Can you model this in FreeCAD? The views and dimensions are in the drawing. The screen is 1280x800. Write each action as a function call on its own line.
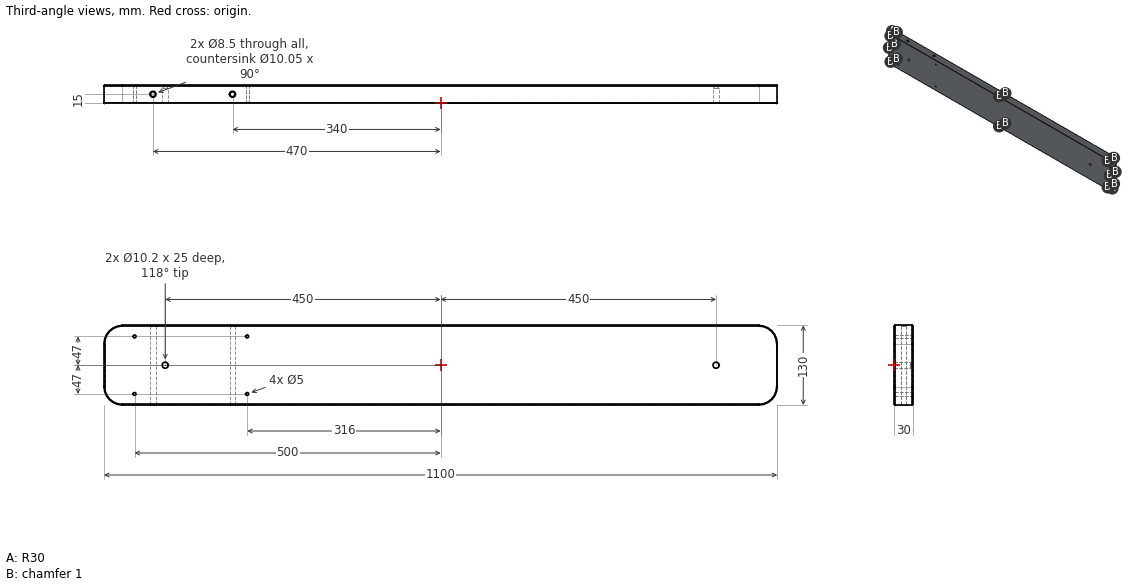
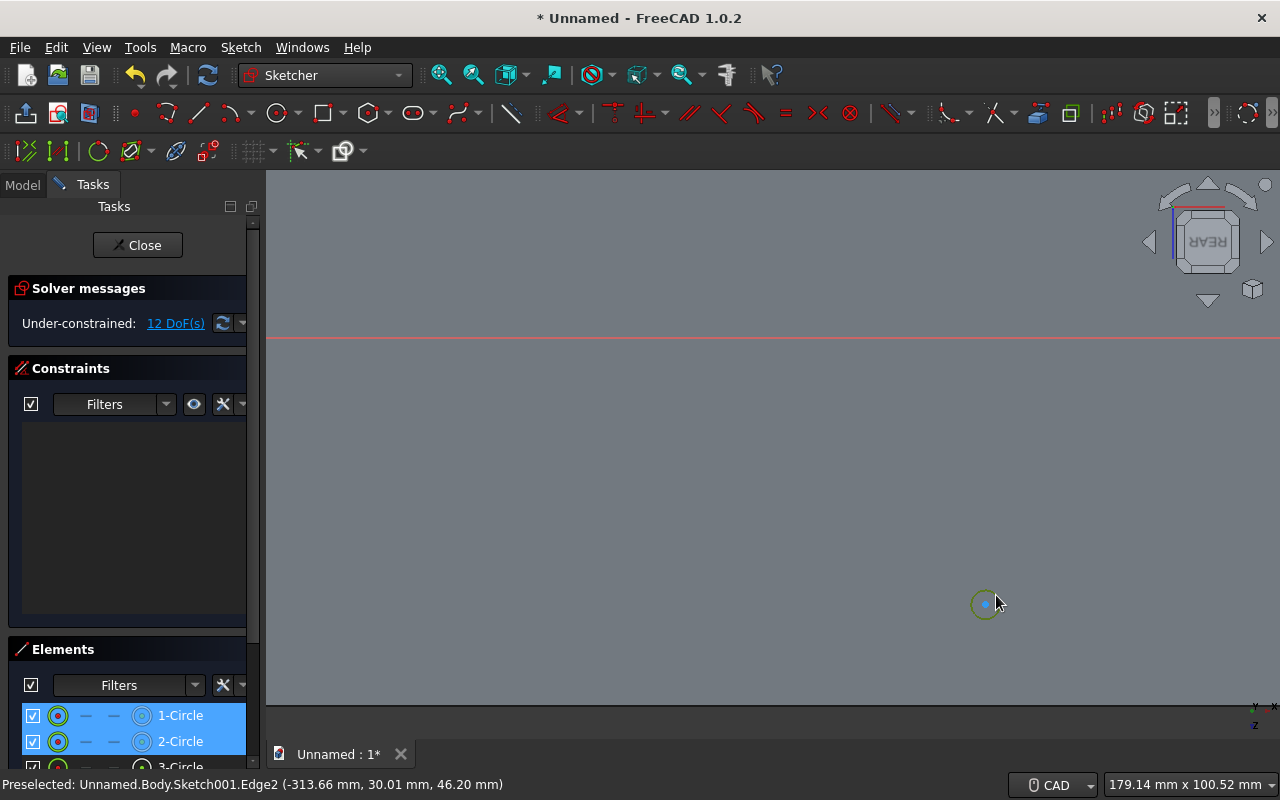
scroll(996, 596, down, 3)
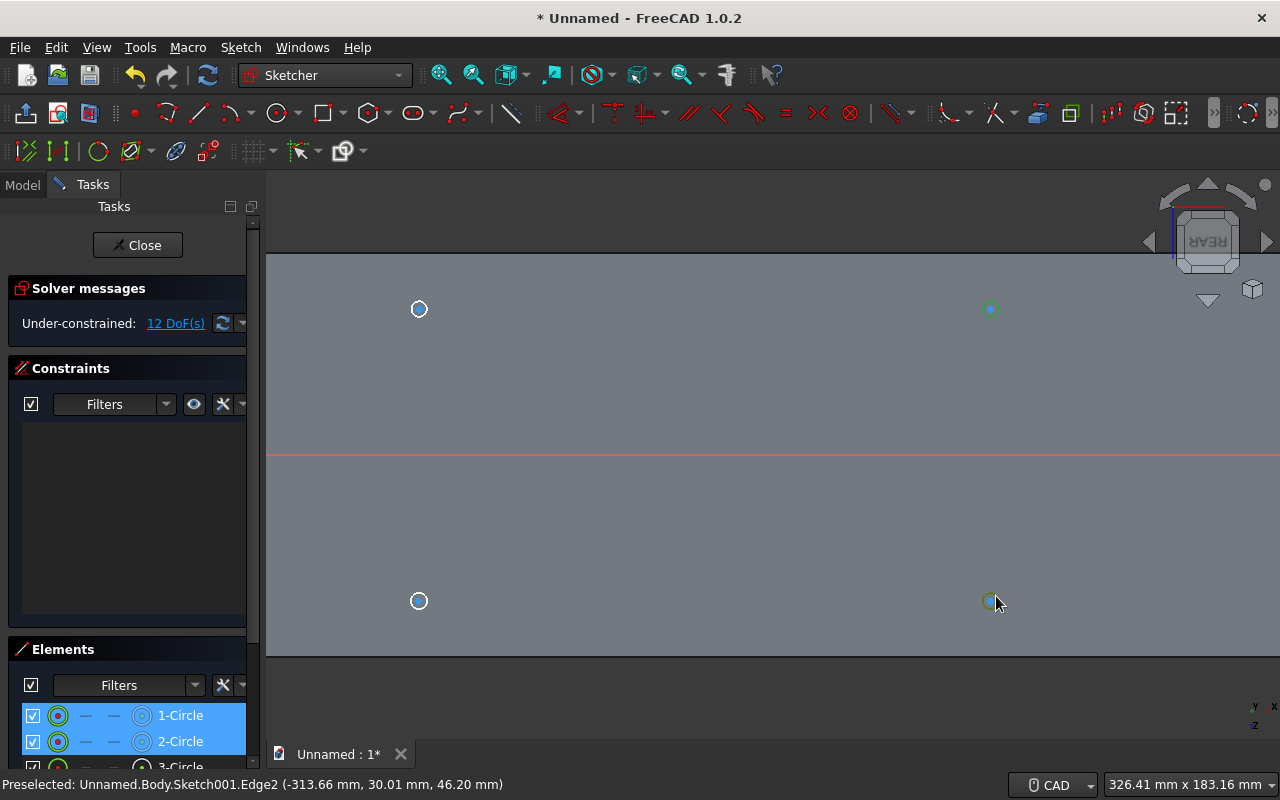
scroll(425, 304, up, 3)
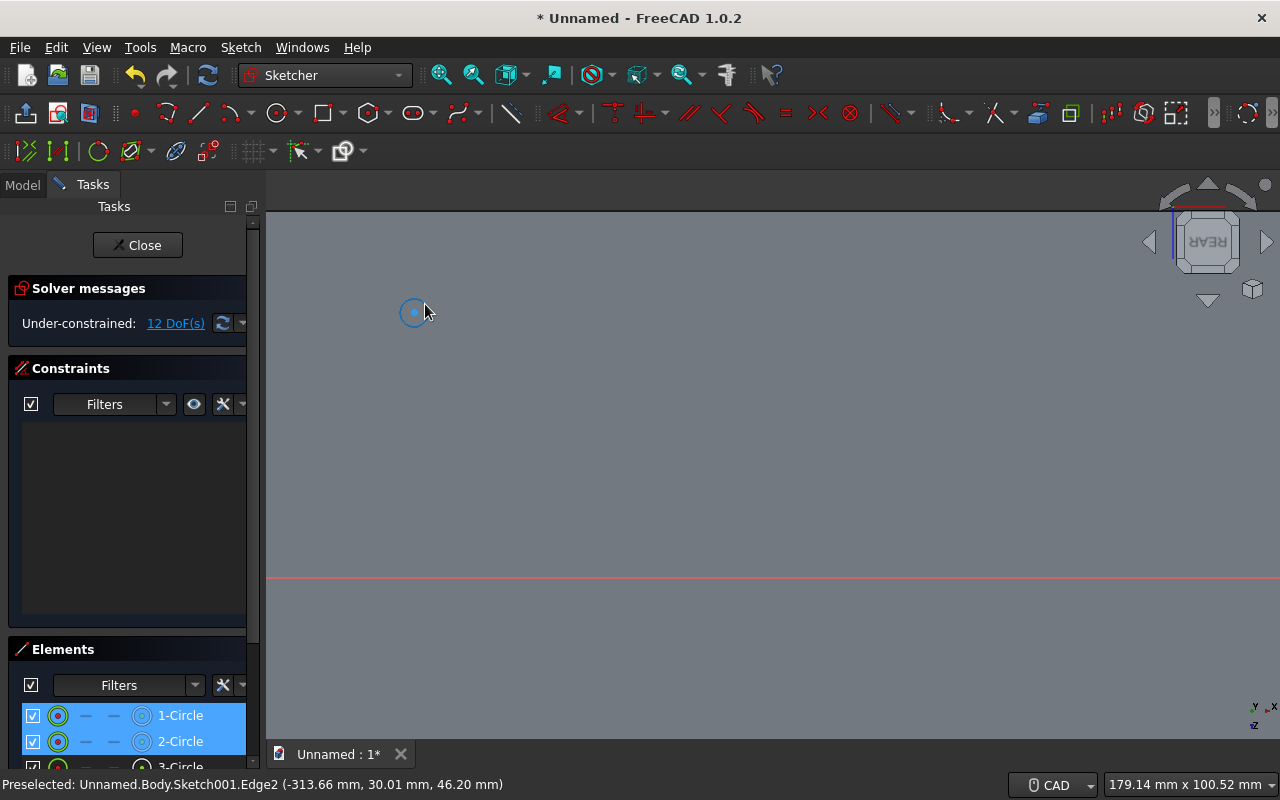
click(424, 303)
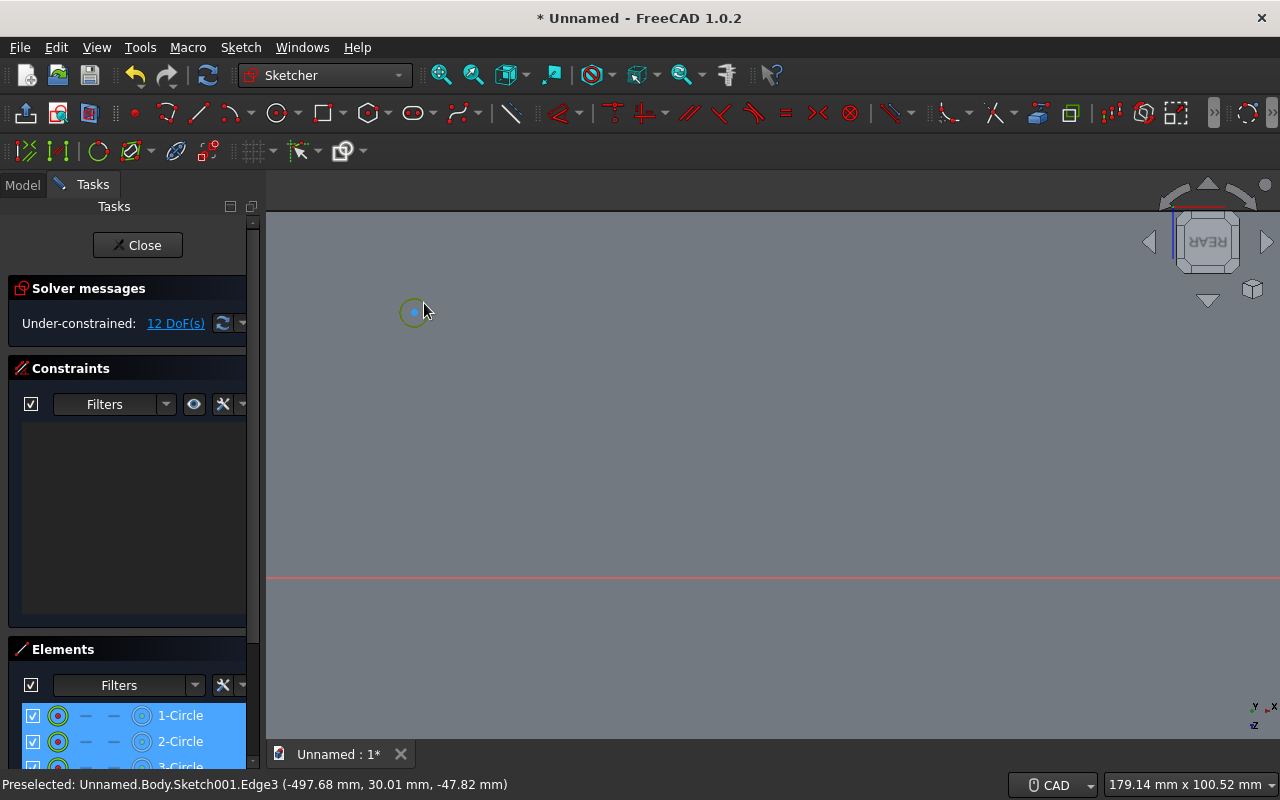
scroll(424, 304, down, 3)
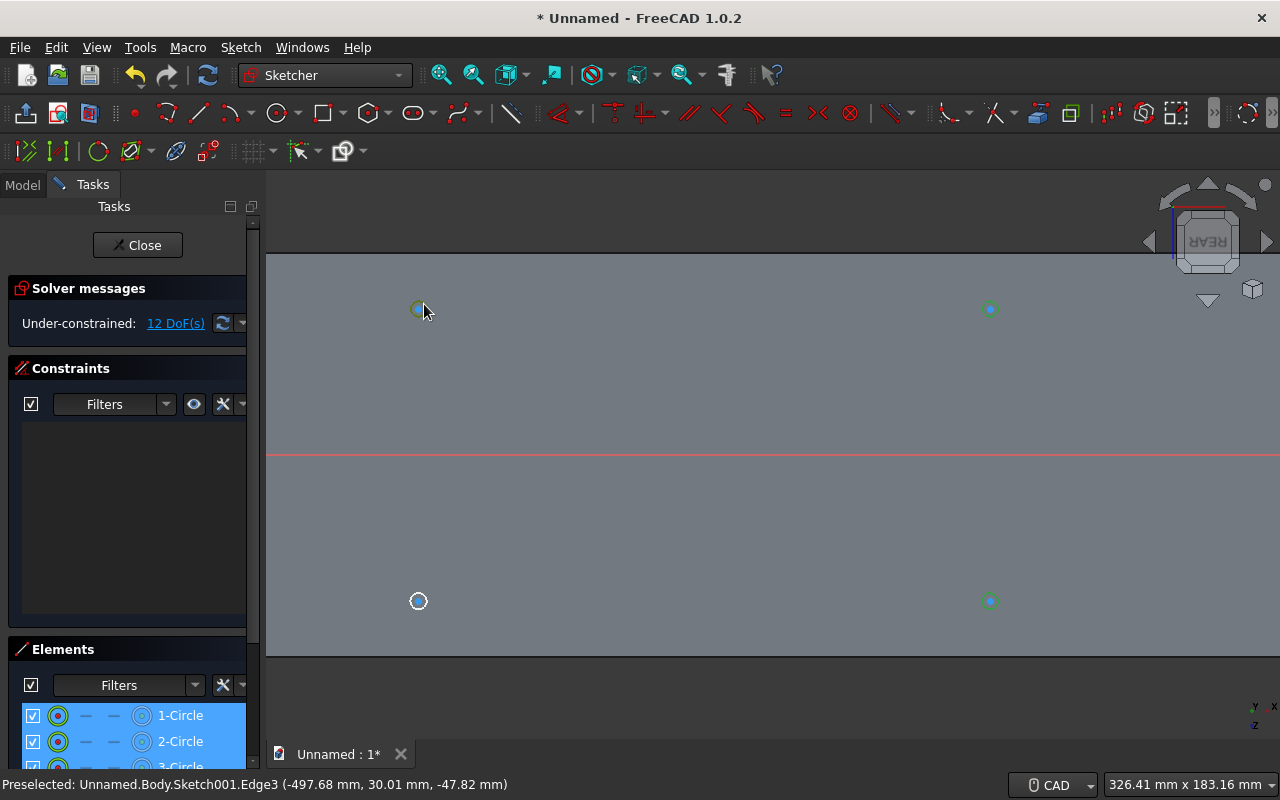
scroll(424, 595, up, 3)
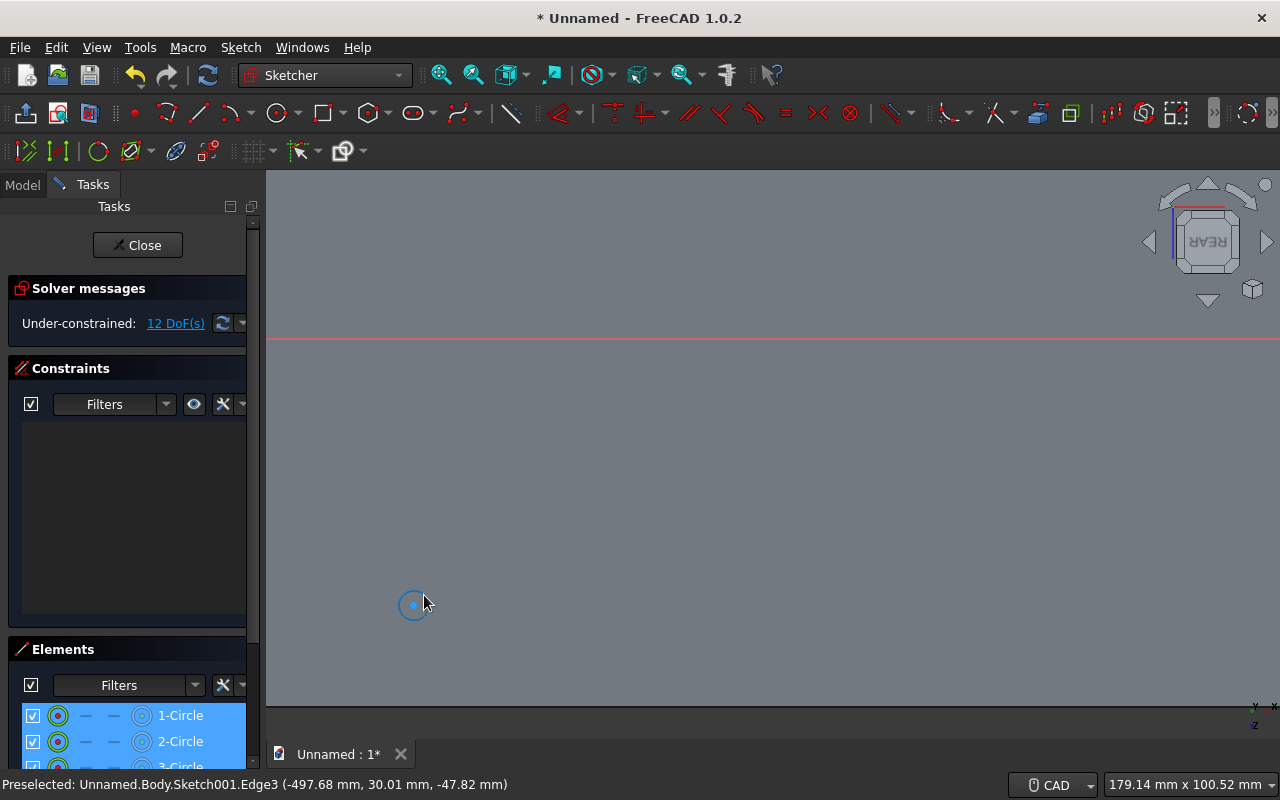
click(424, 595)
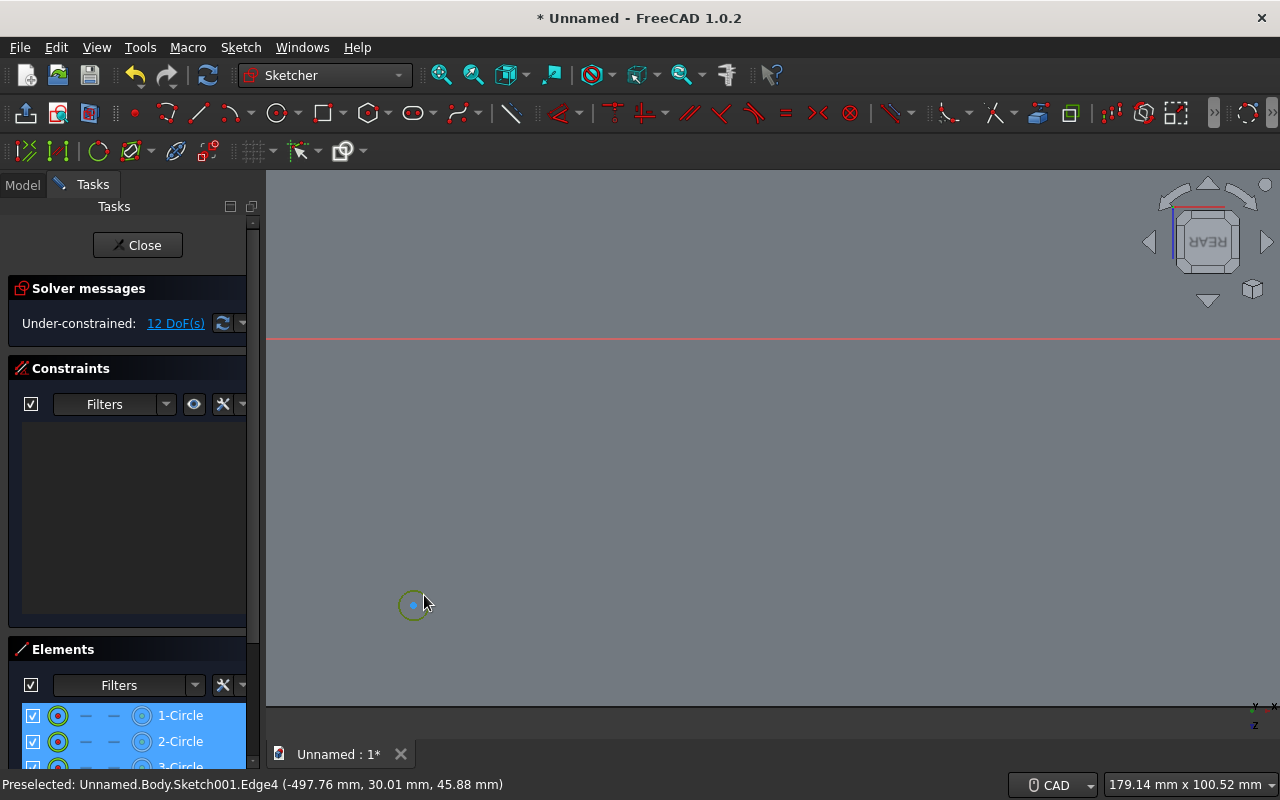
click(786, 114)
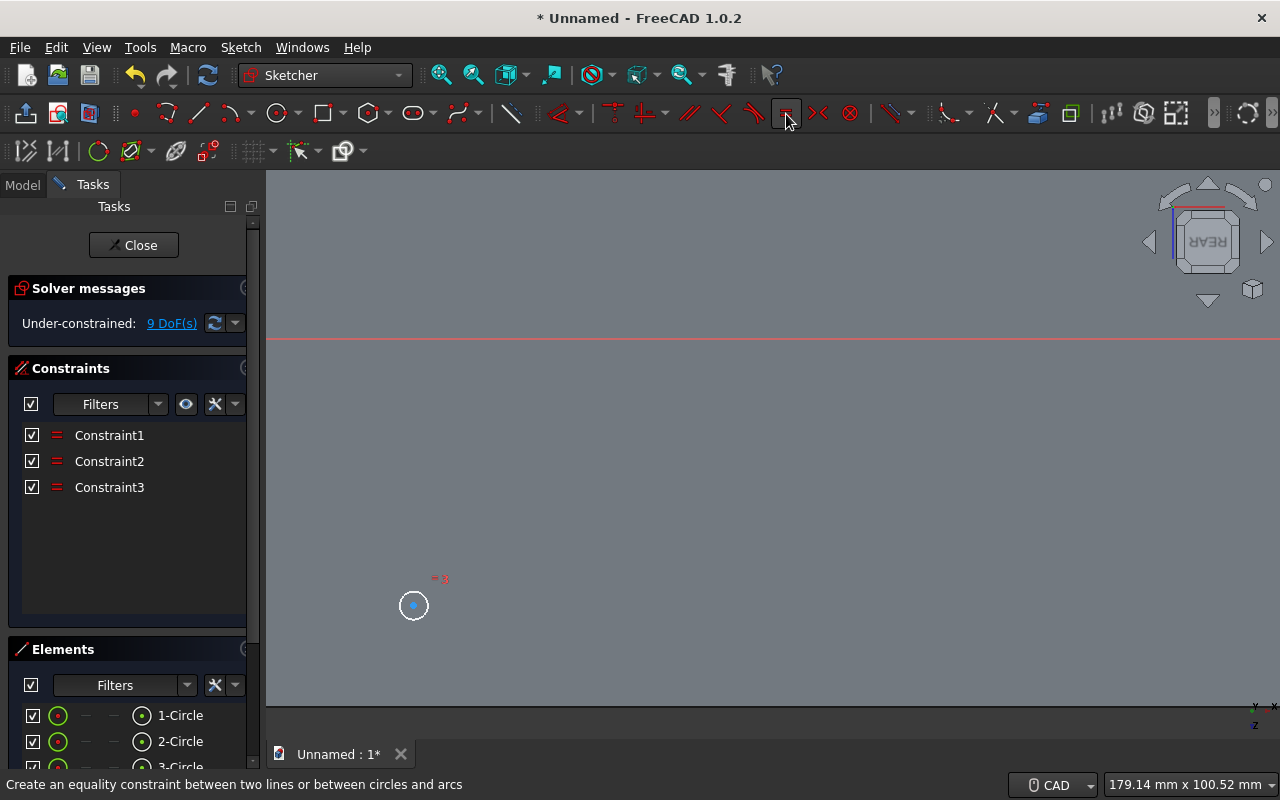
scroll(424, 595, down, 3)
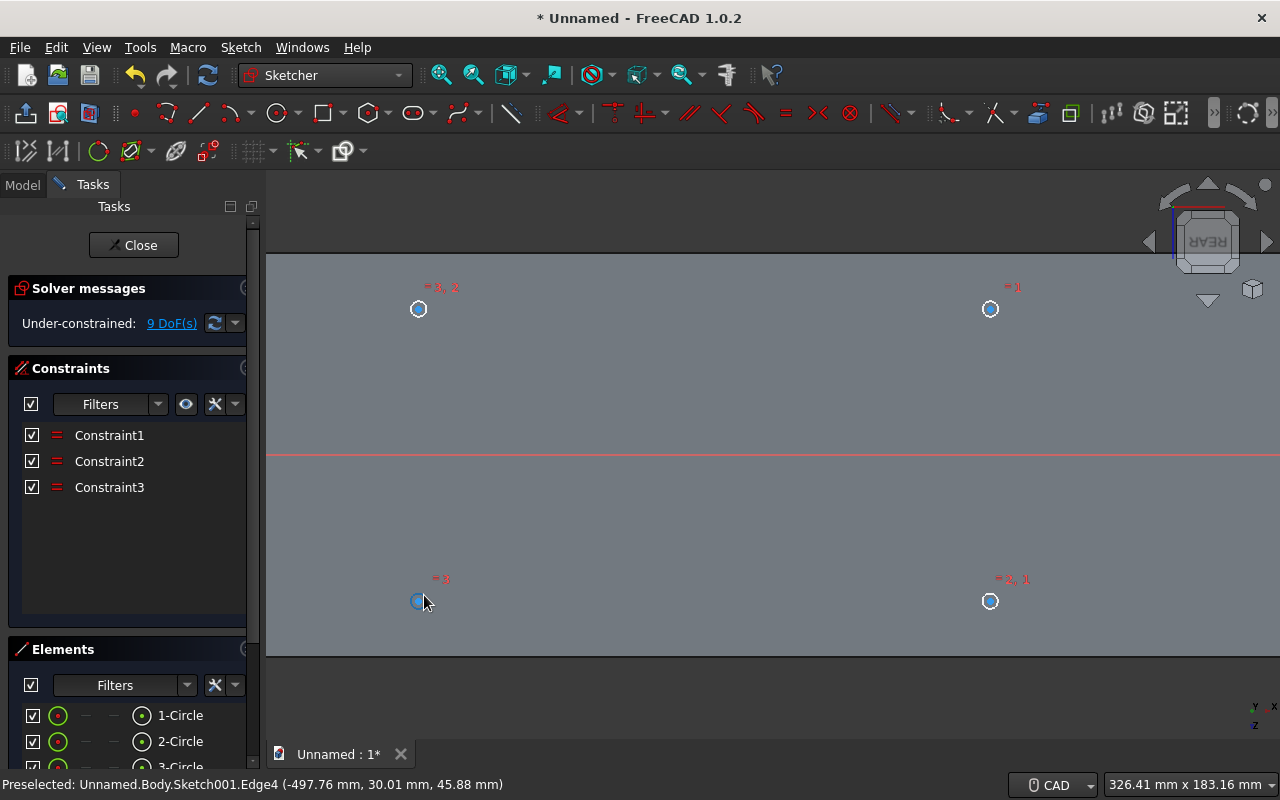
click(990, 309)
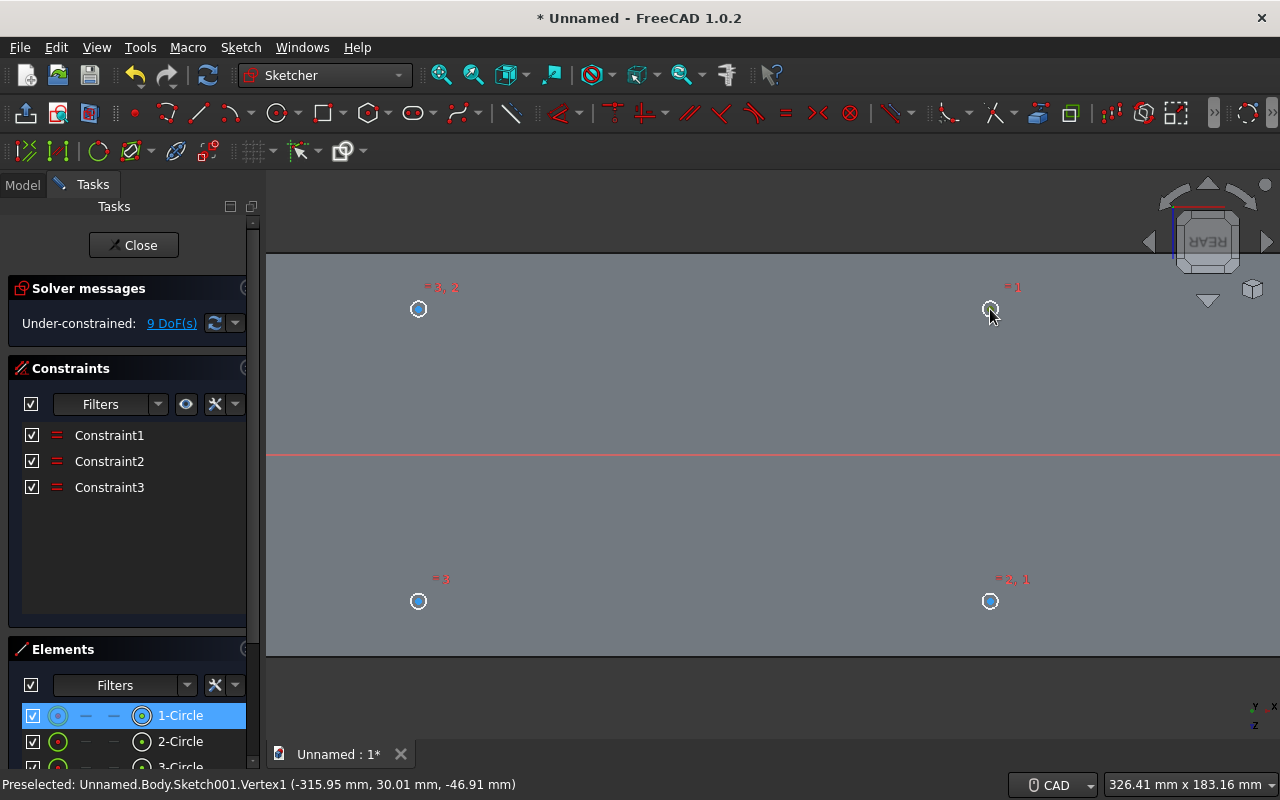
click(990, 601)